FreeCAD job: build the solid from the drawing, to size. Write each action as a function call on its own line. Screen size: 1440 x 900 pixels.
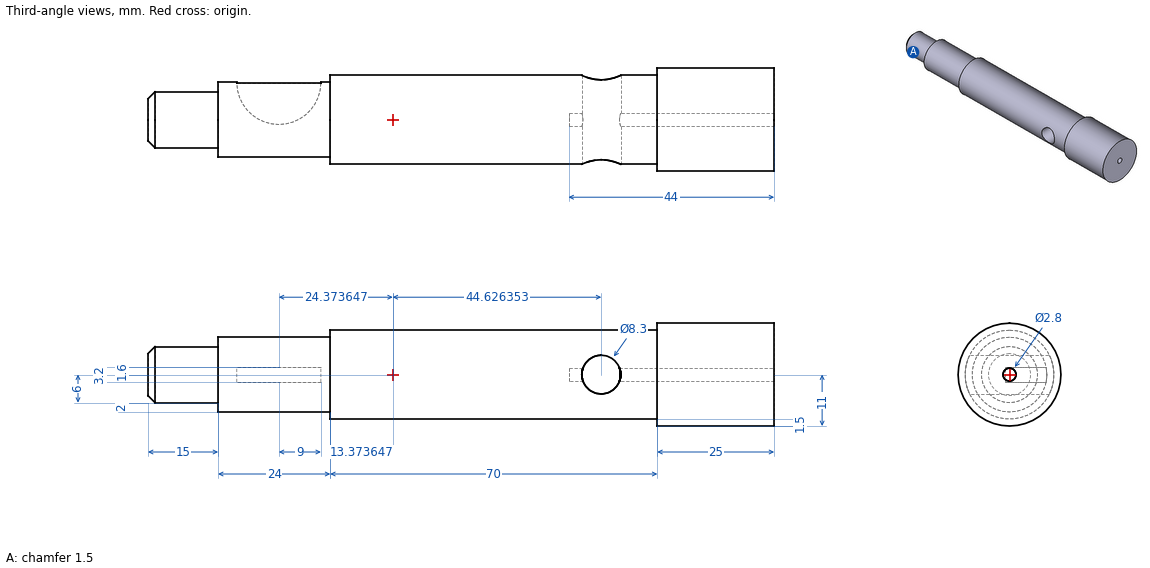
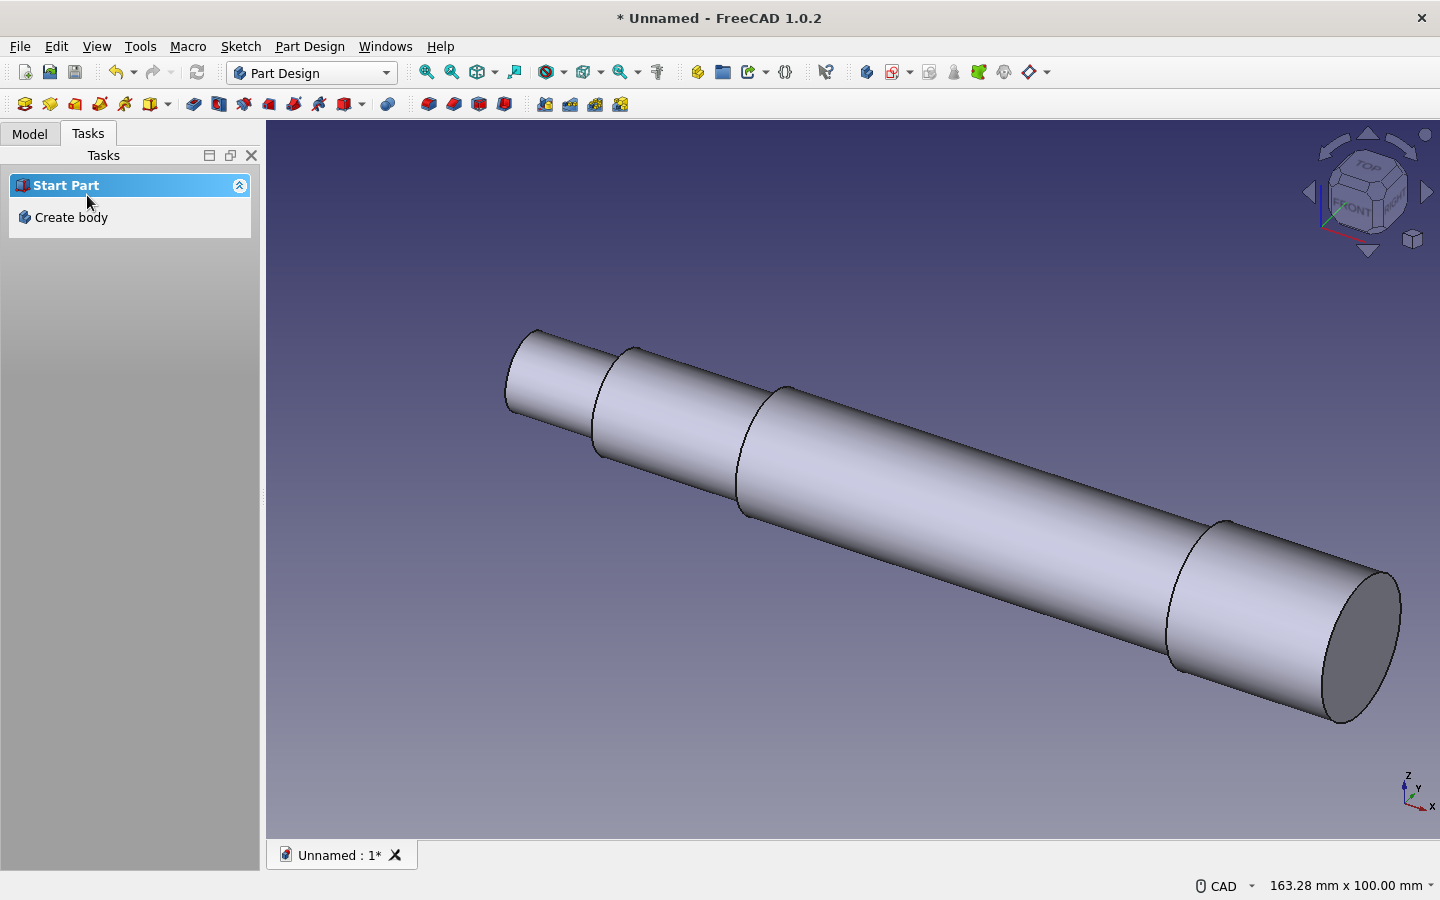
click(1361, 647)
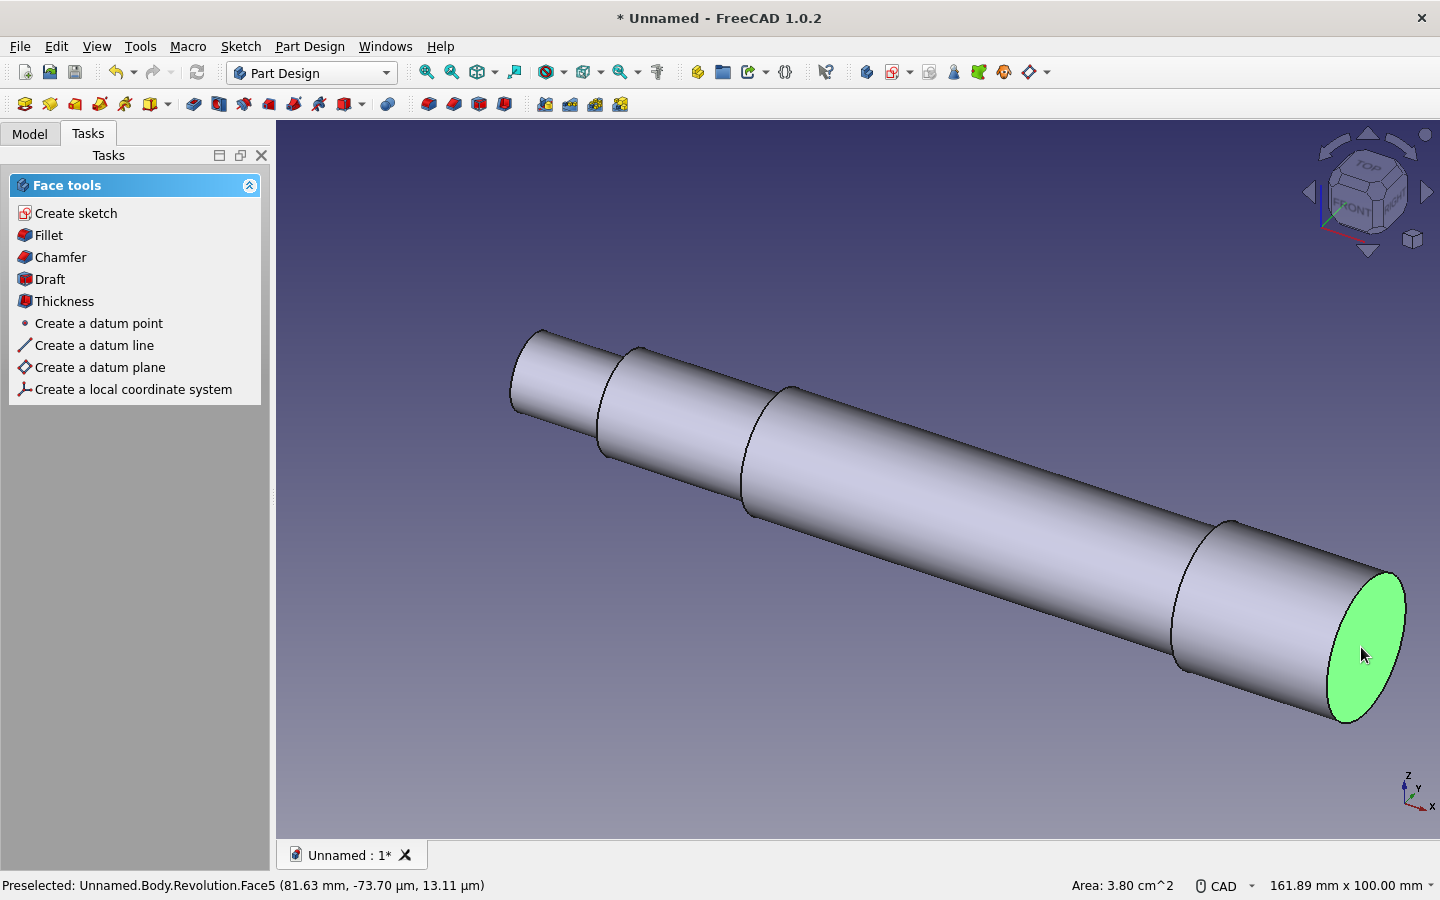
click(892, 72)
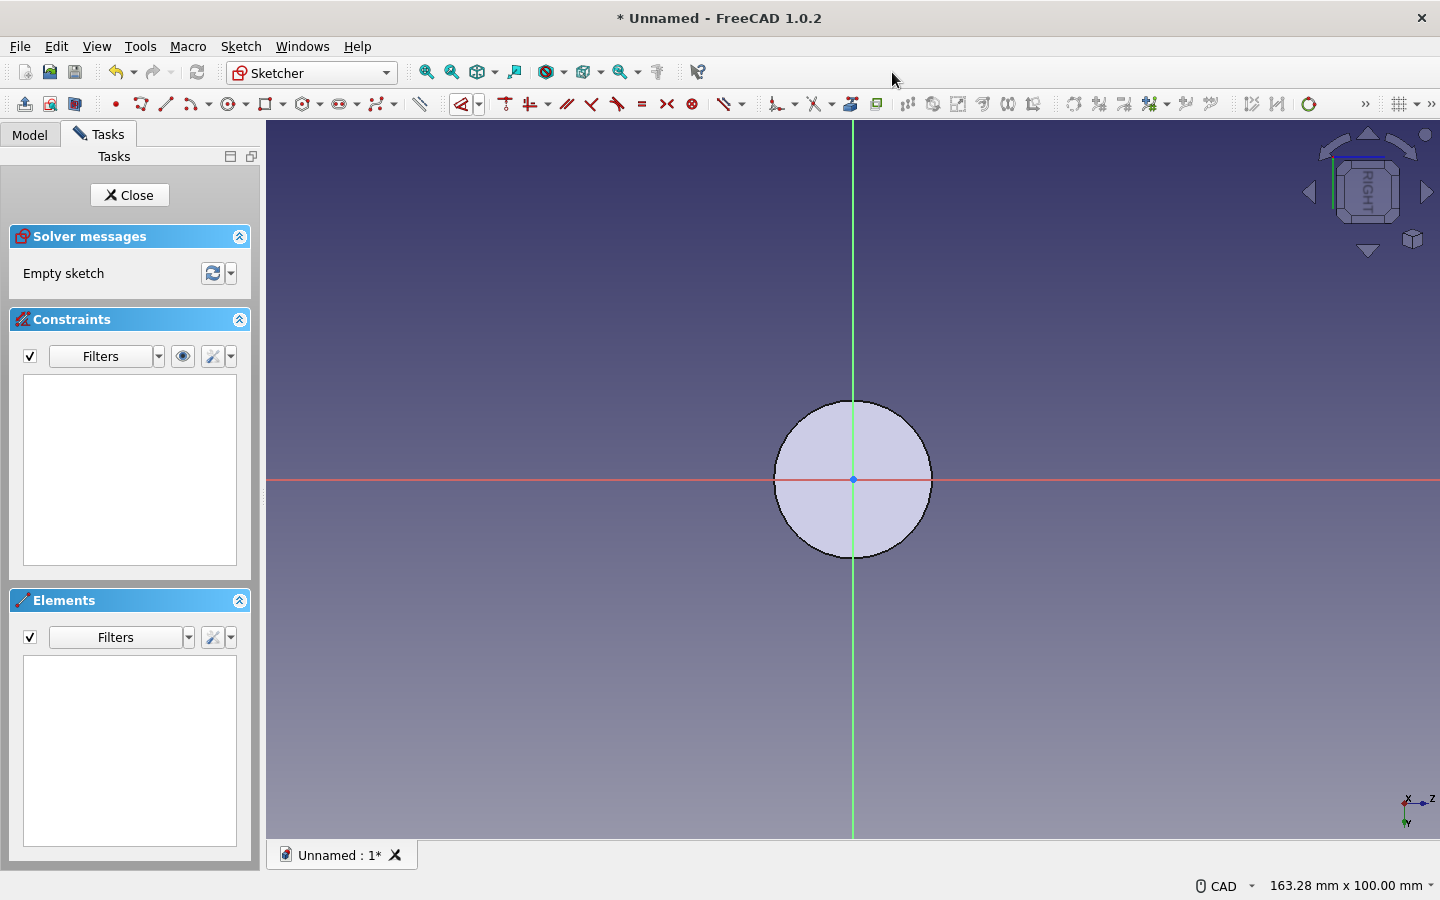
scroll(857, 479, up, 15)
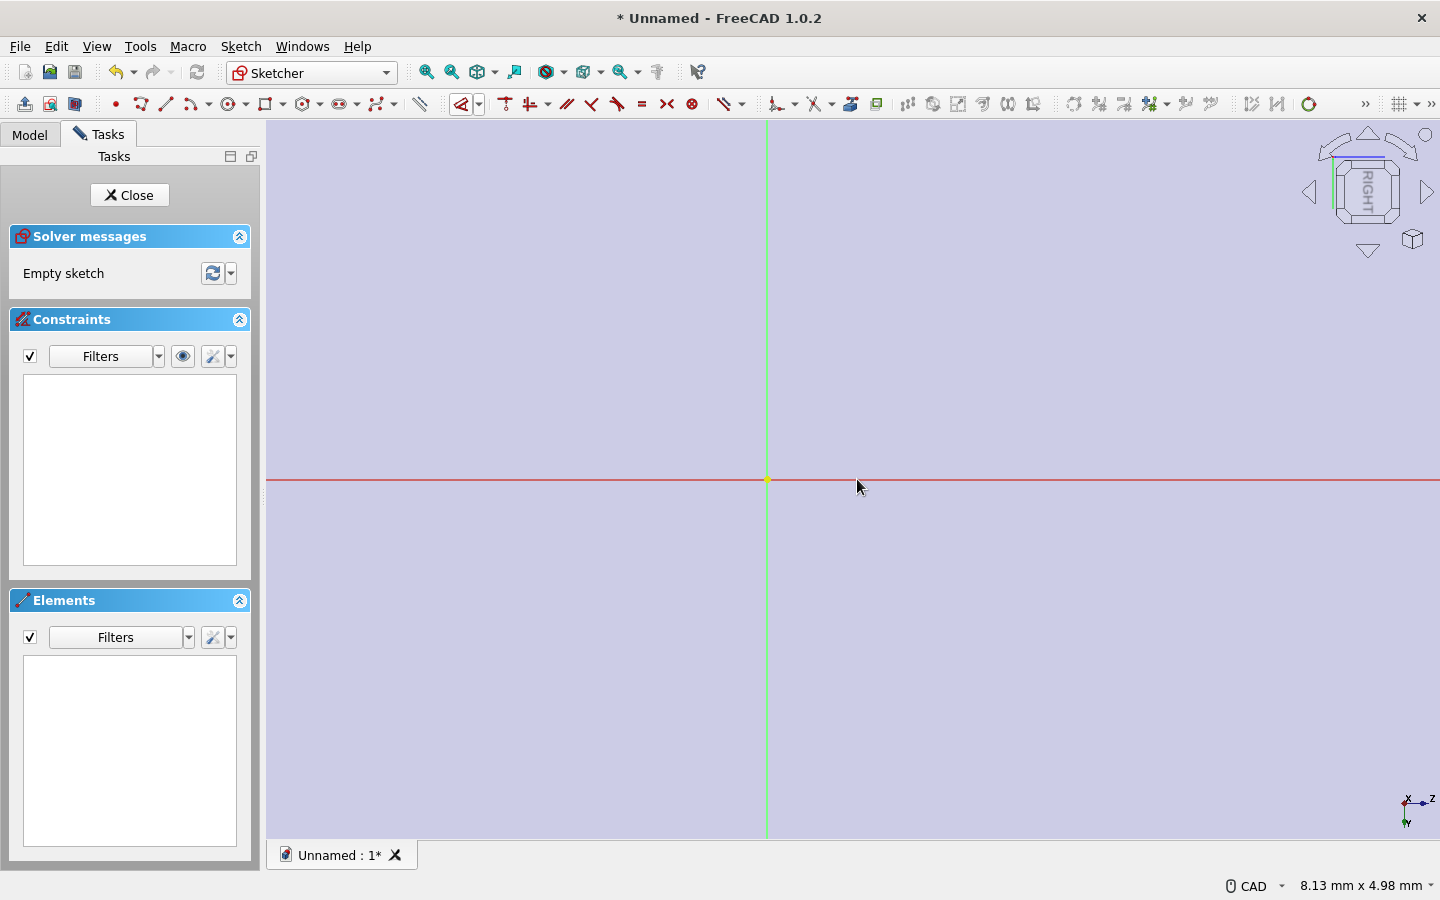
click(228, 104)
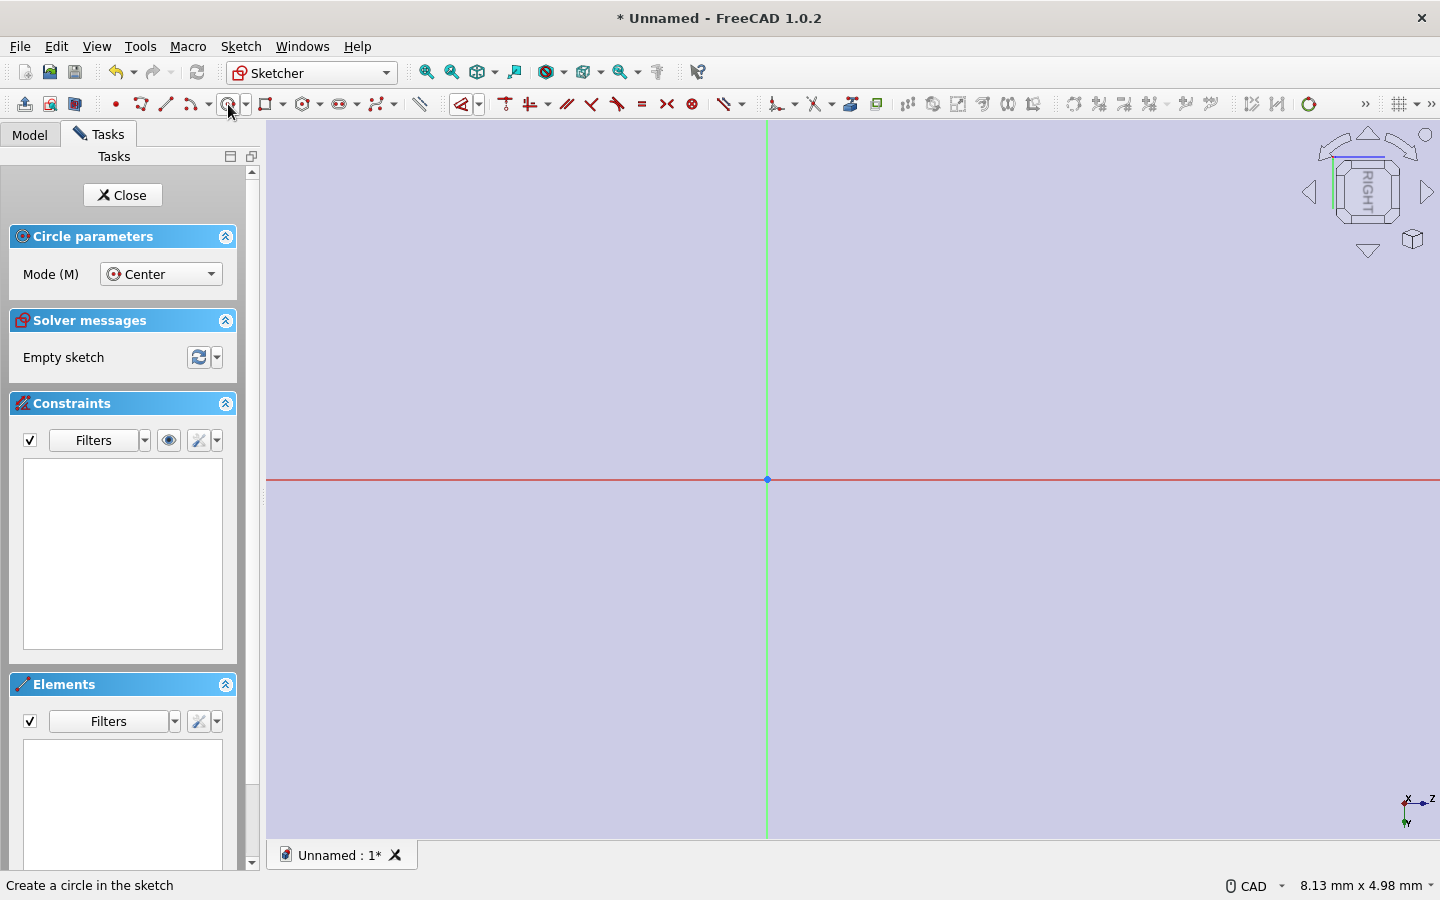
click(767, 480)
click(910, 337)
key(Escape)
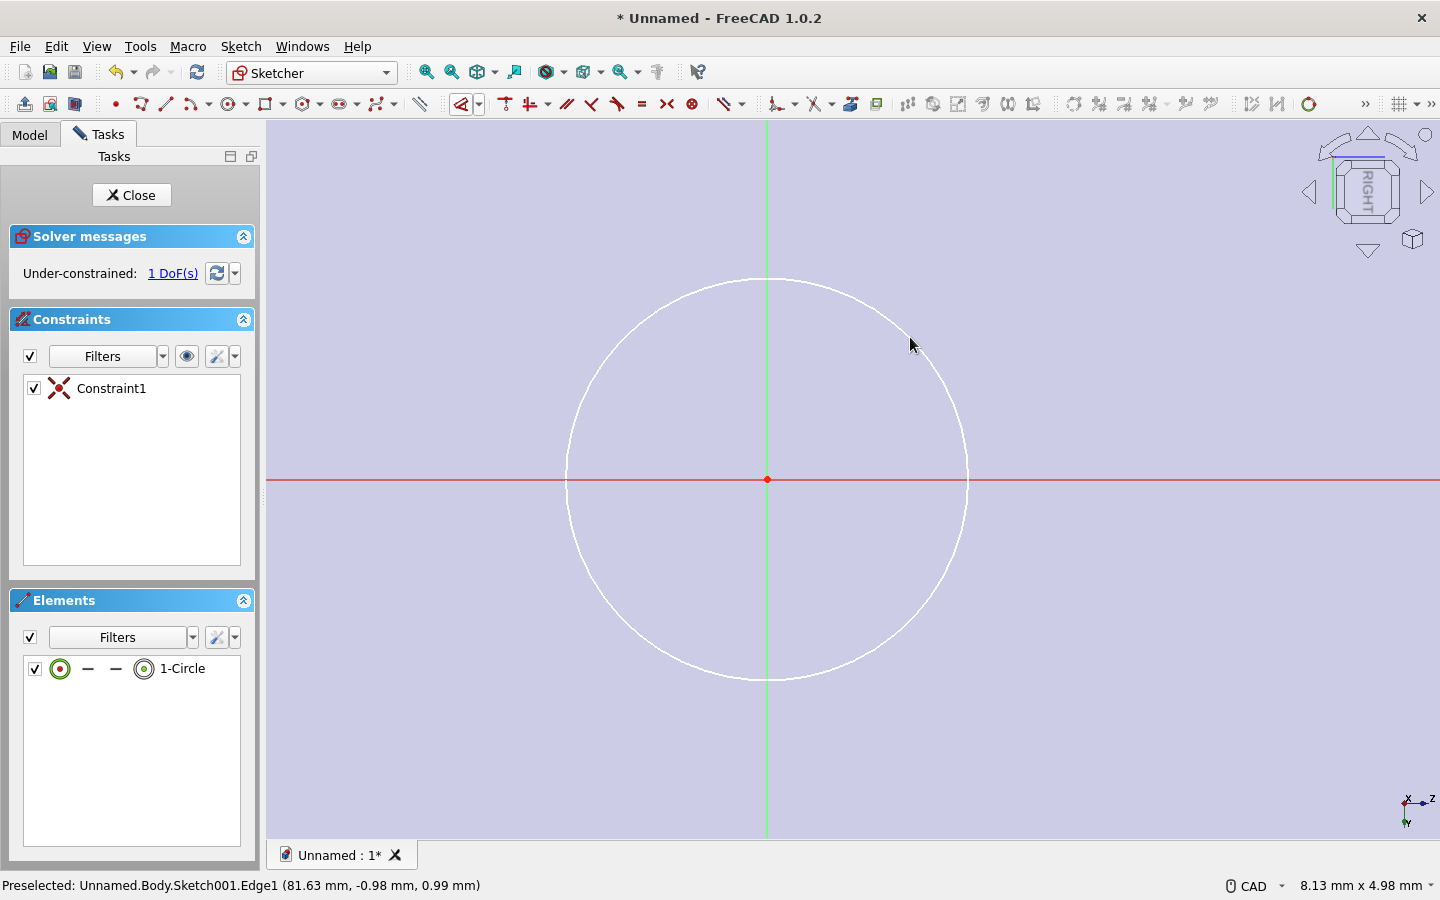
click(909, 337)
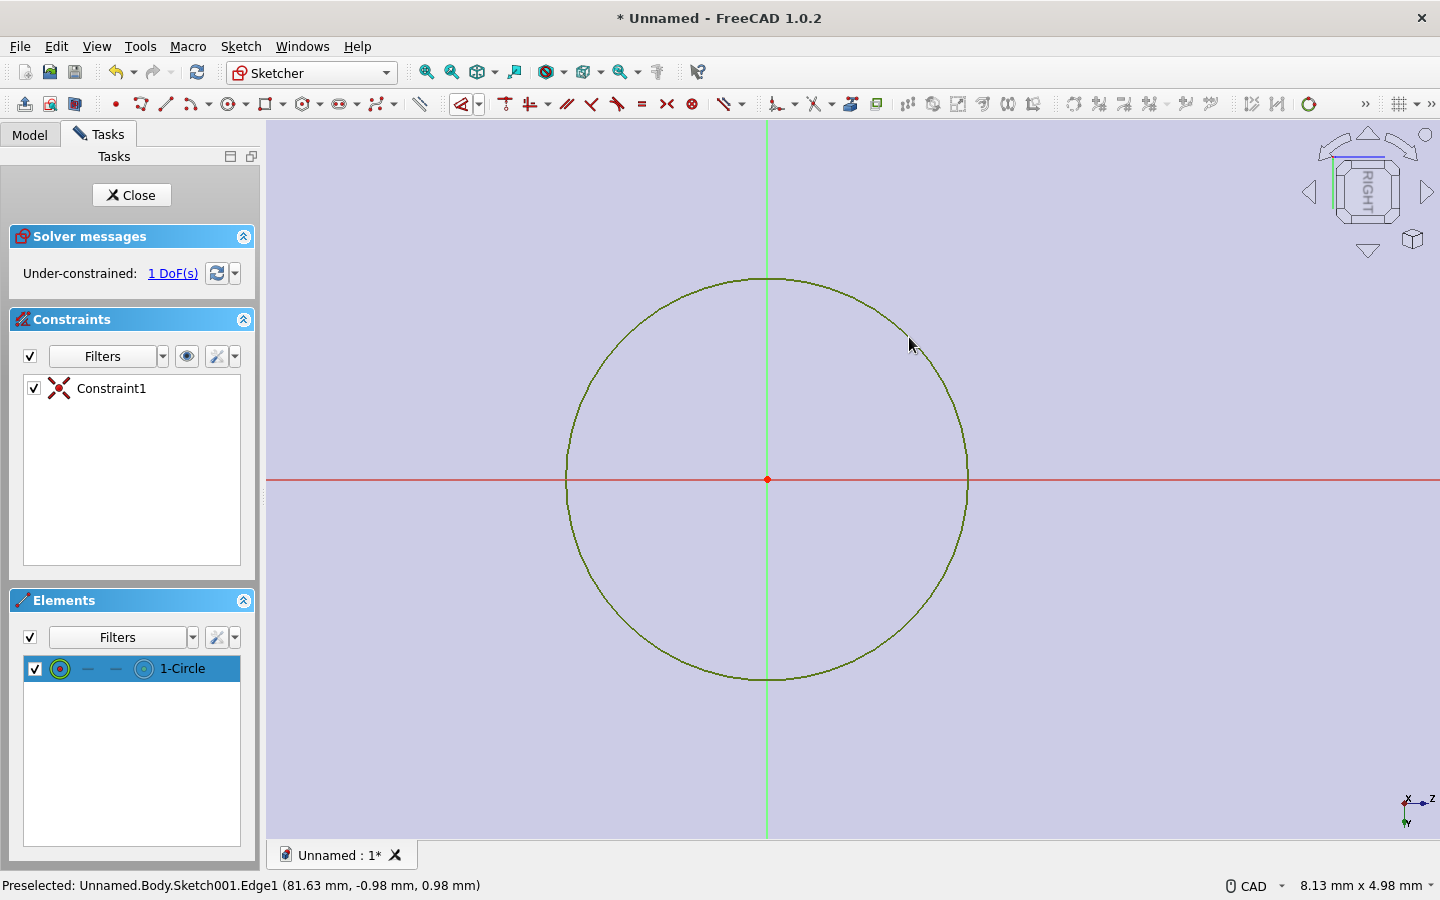
click(478, 104)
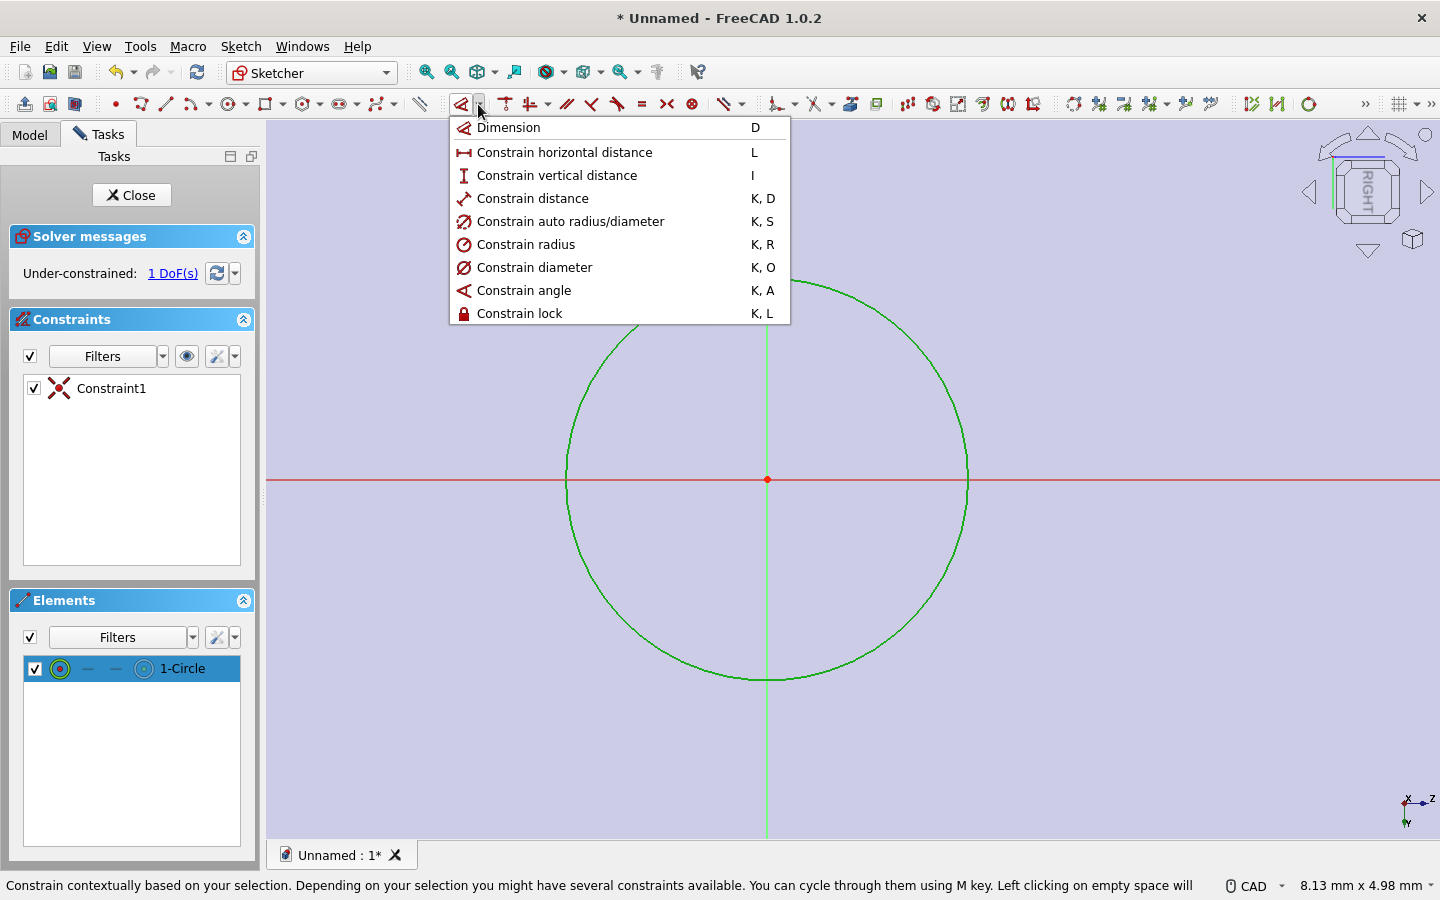
click(620, 268)